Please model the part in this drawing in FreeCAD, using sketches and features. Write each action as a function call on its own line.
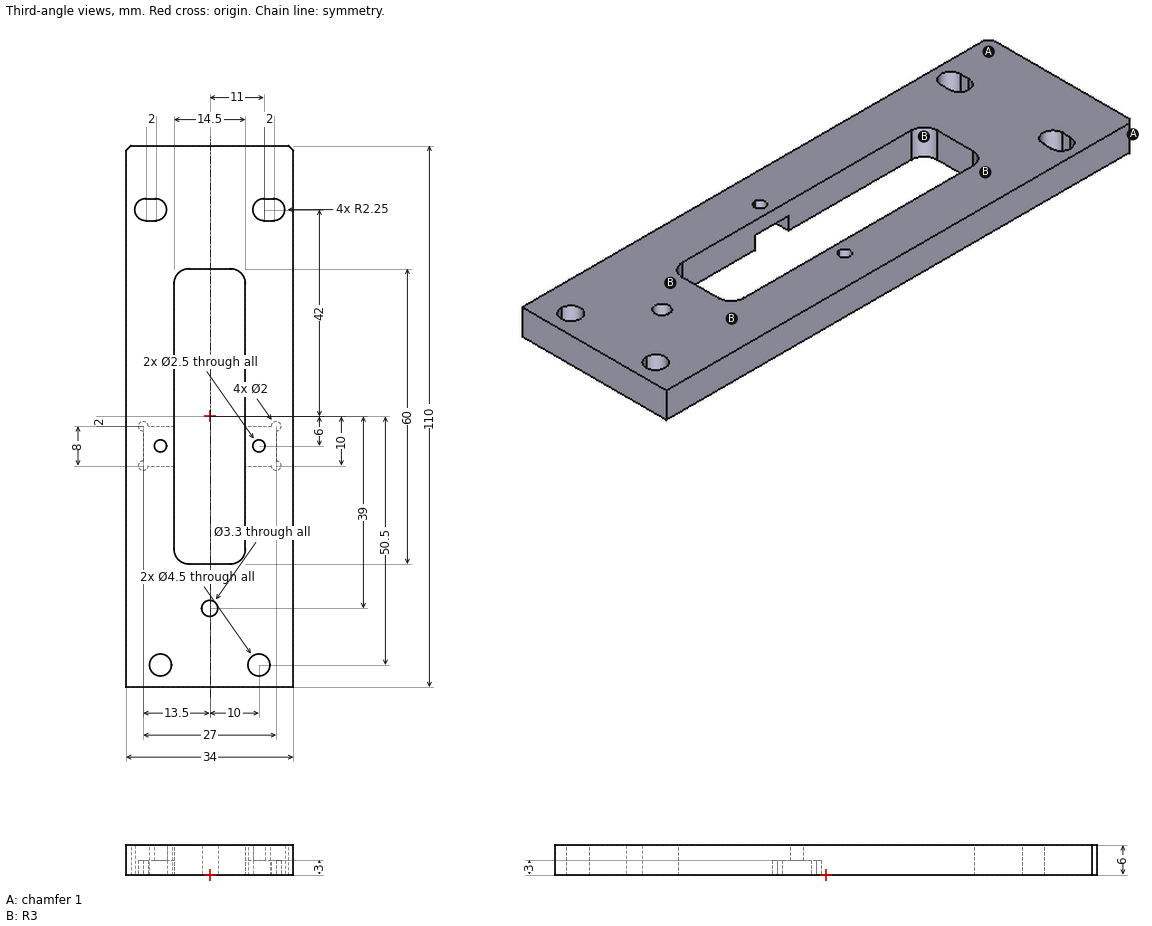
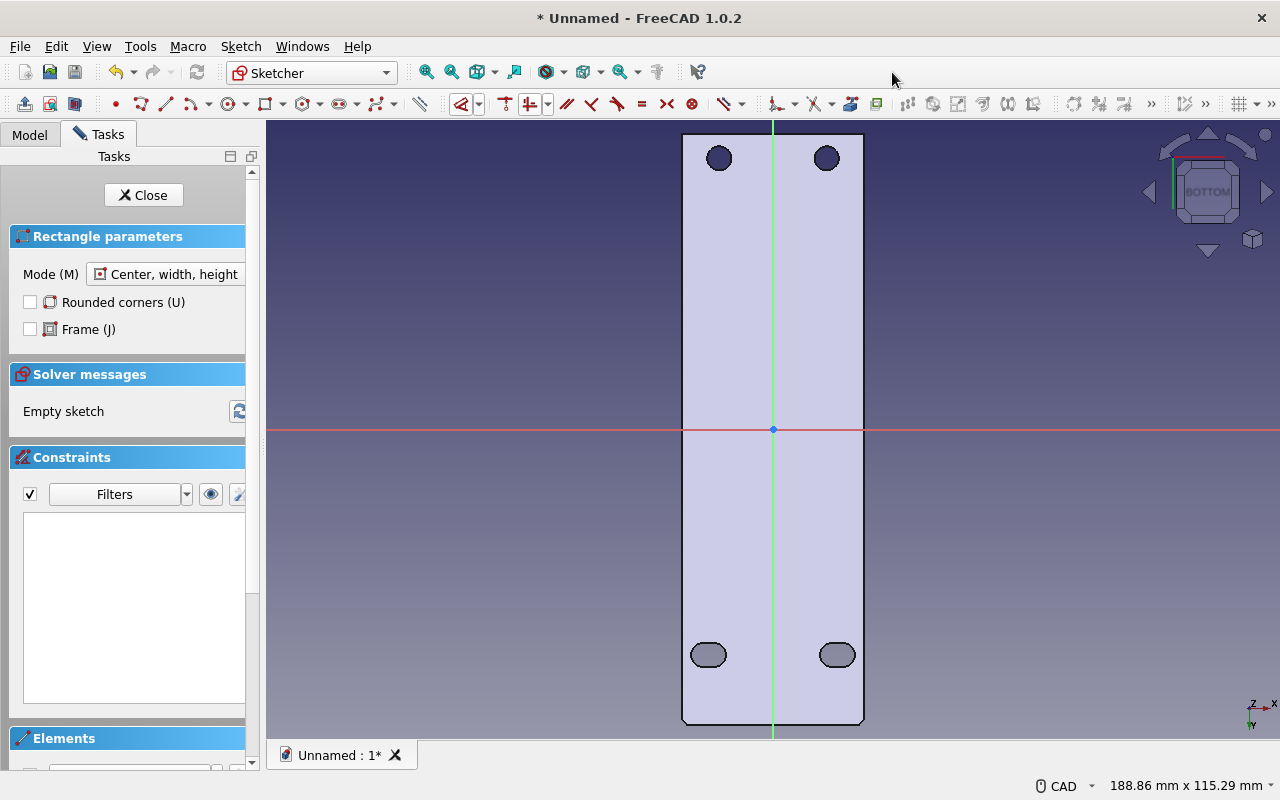
click(773, 430)
click(812, 268)
key(Escape)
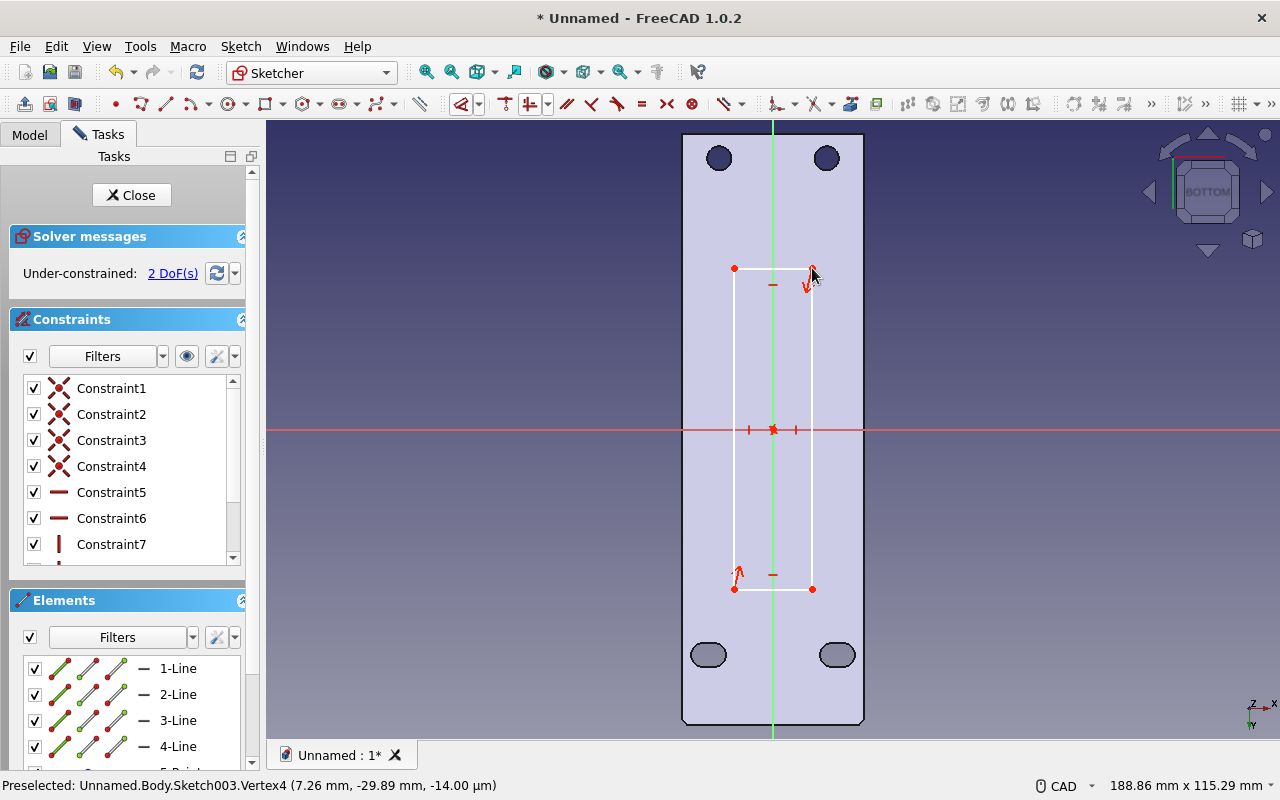
click(812, 494)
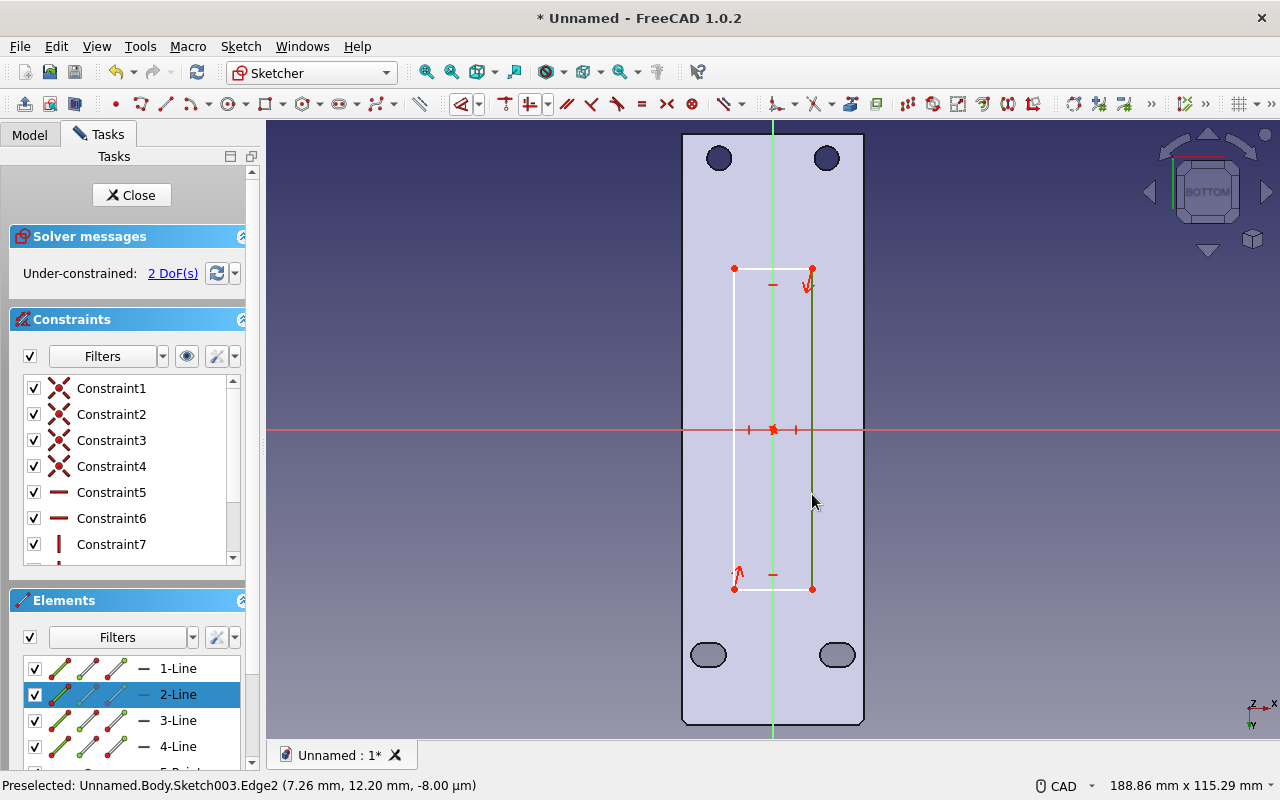
key(i)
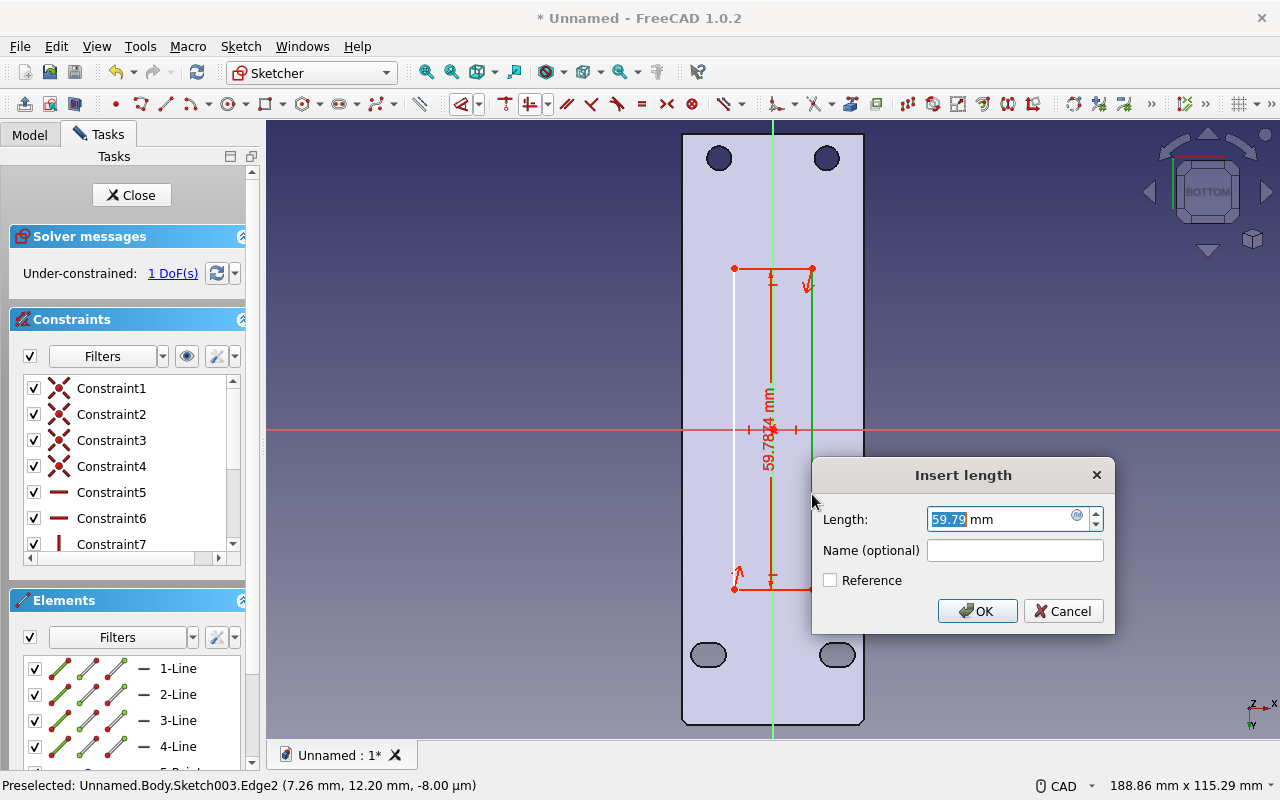
text(60)
key(Return)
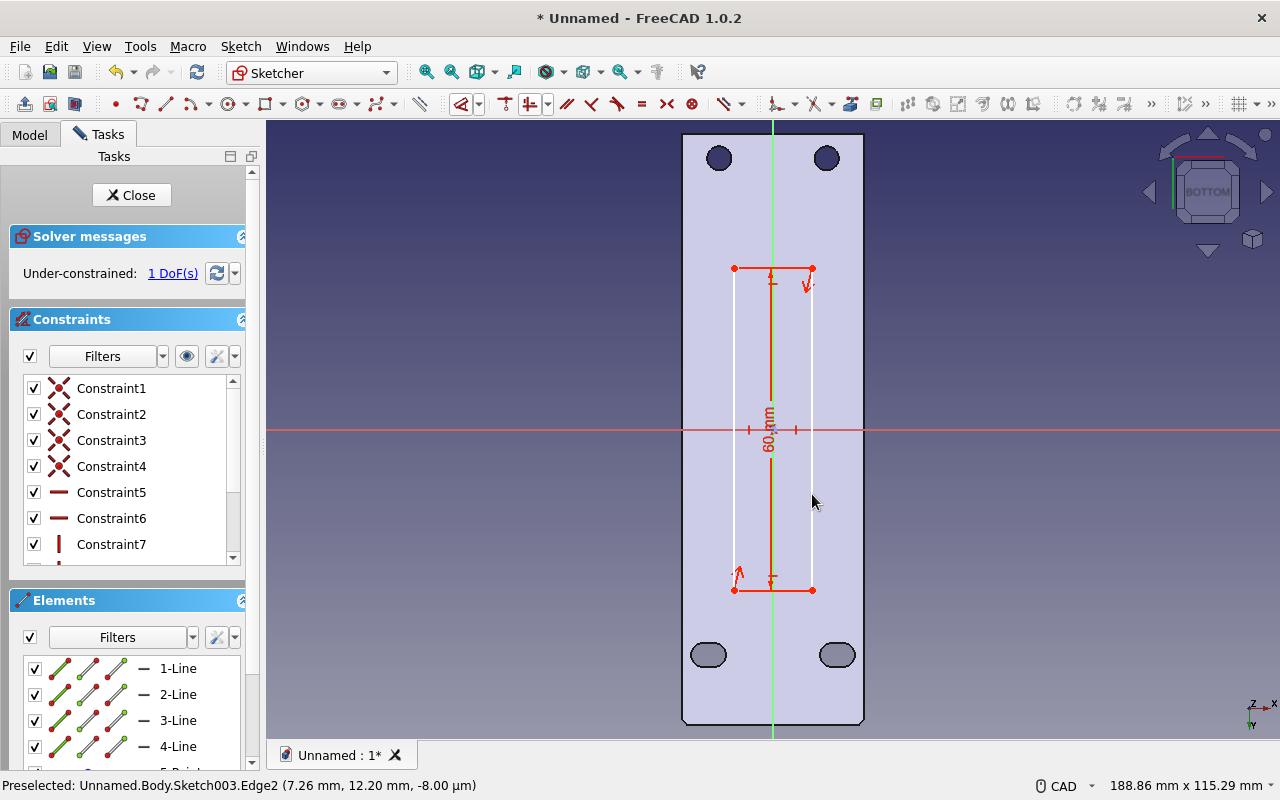
click(757, 591)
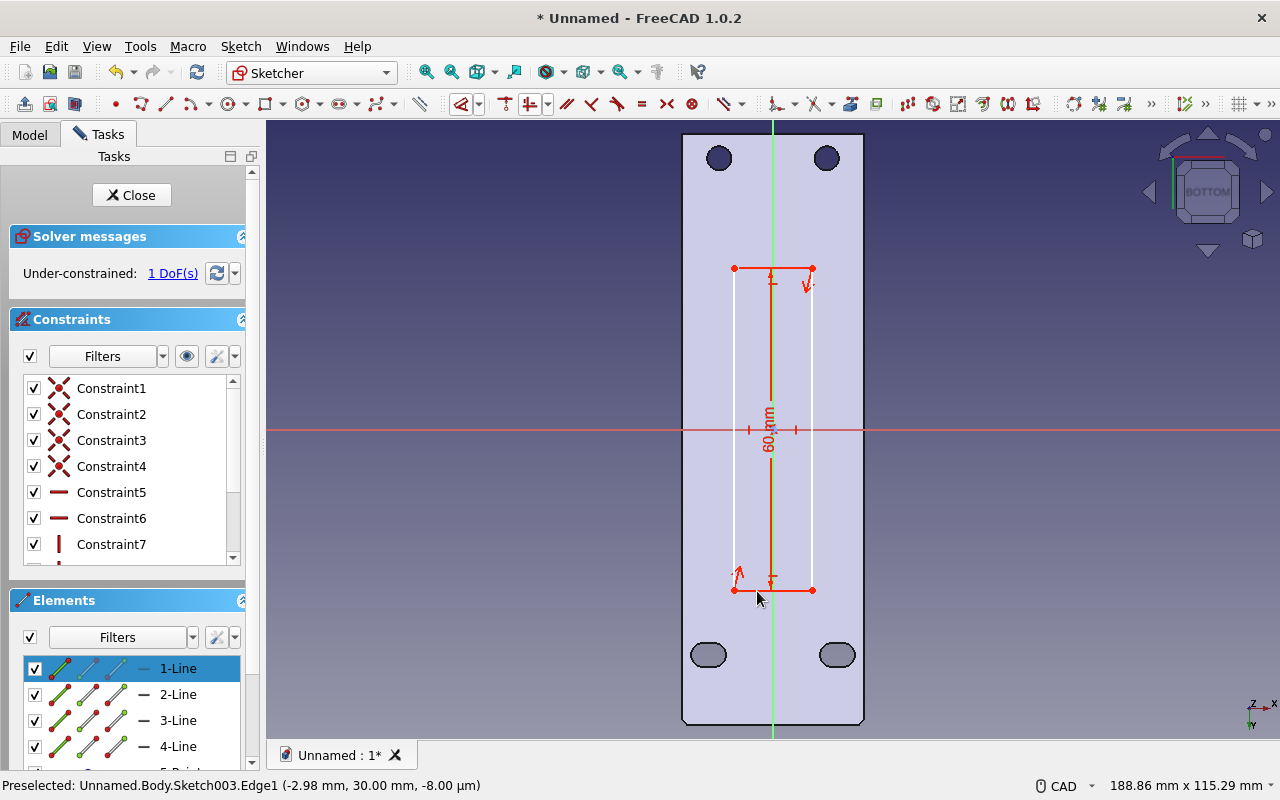
click(478, 104)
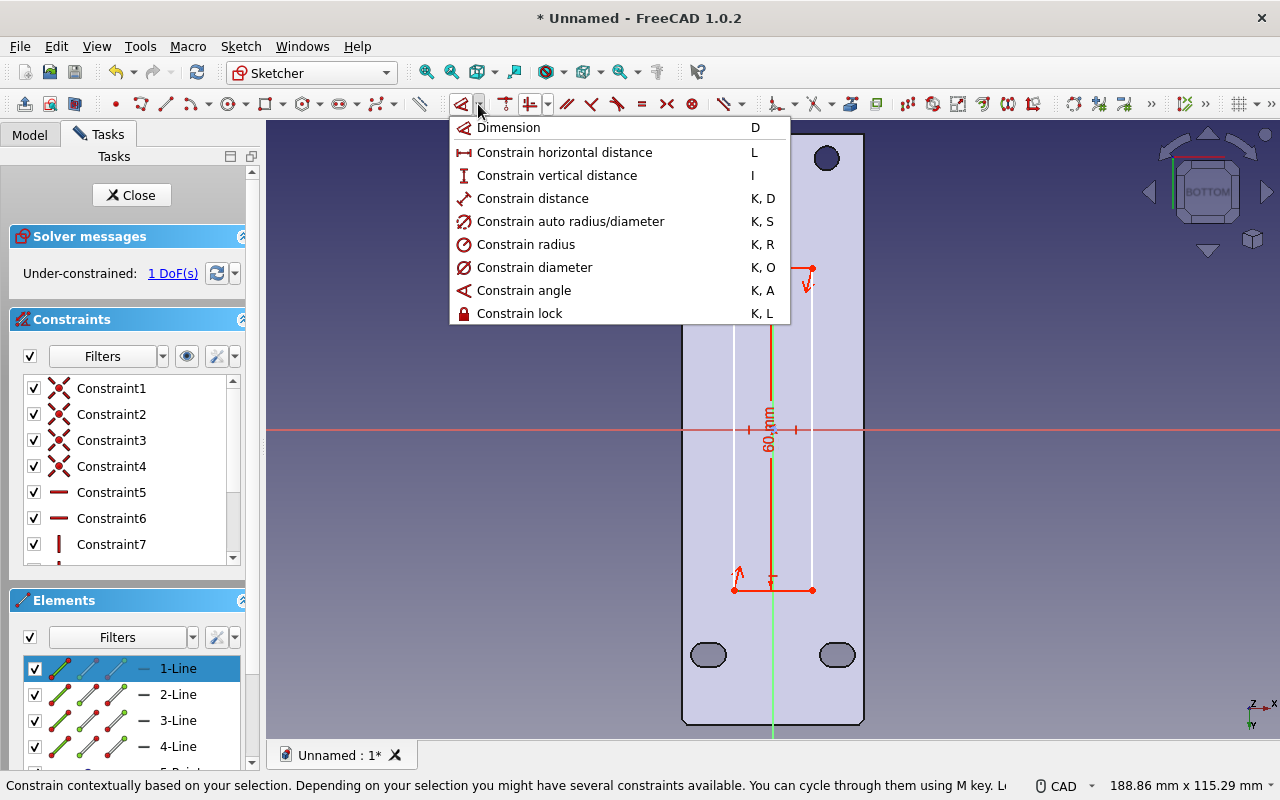
click(620, 152)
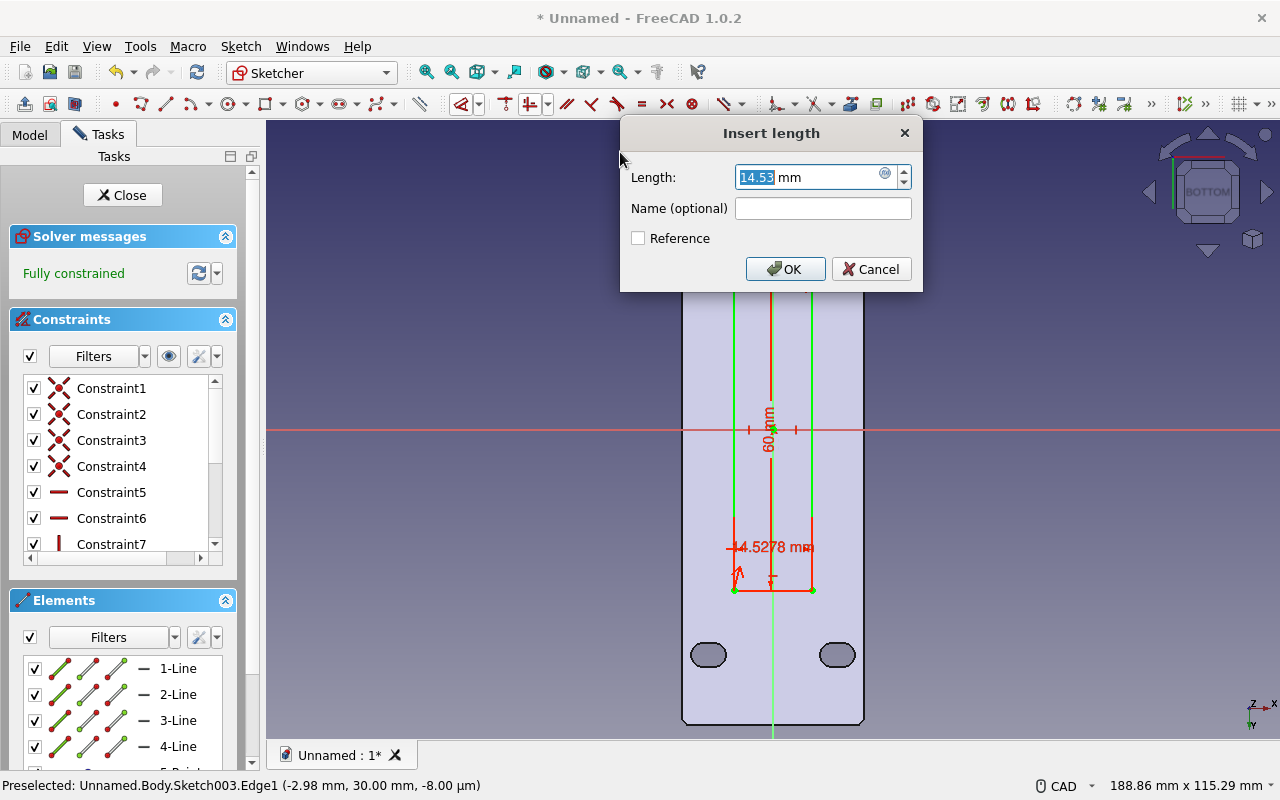
text(14.5)
key(Return)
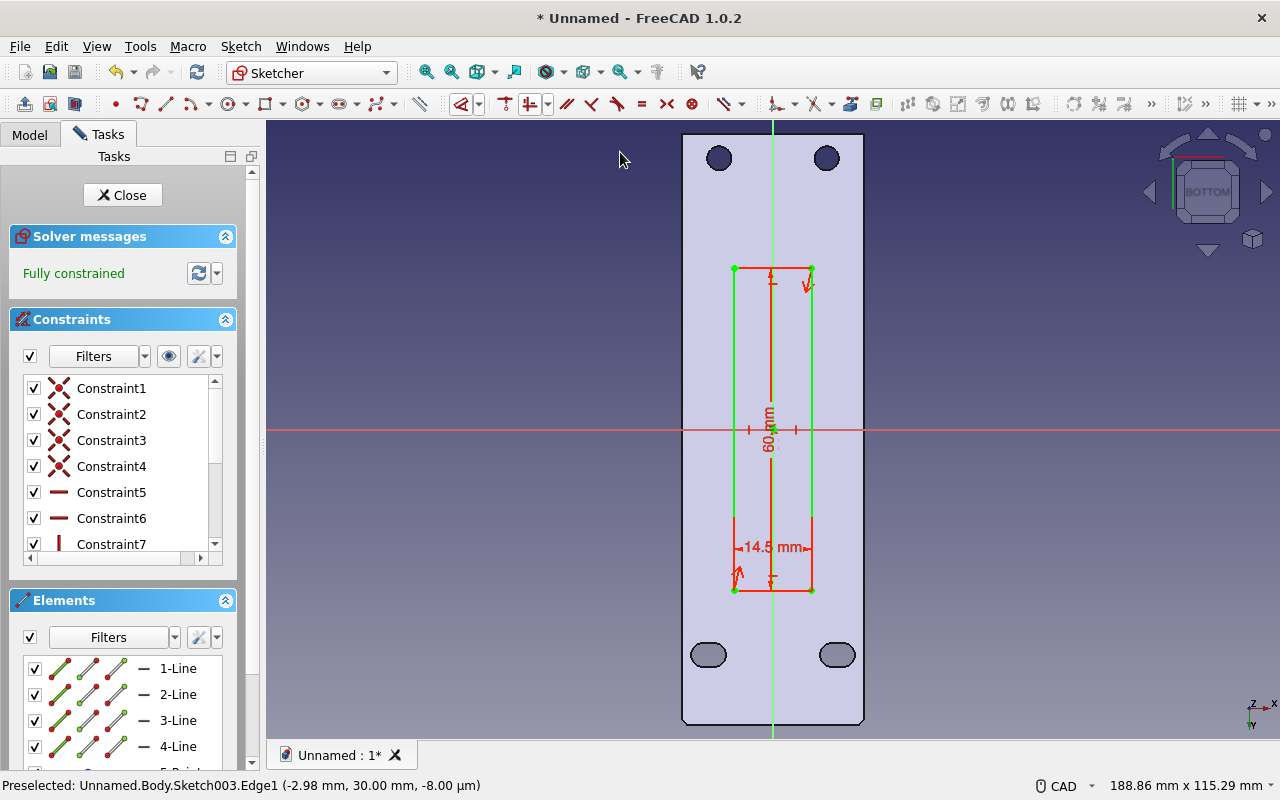
click(123, 195)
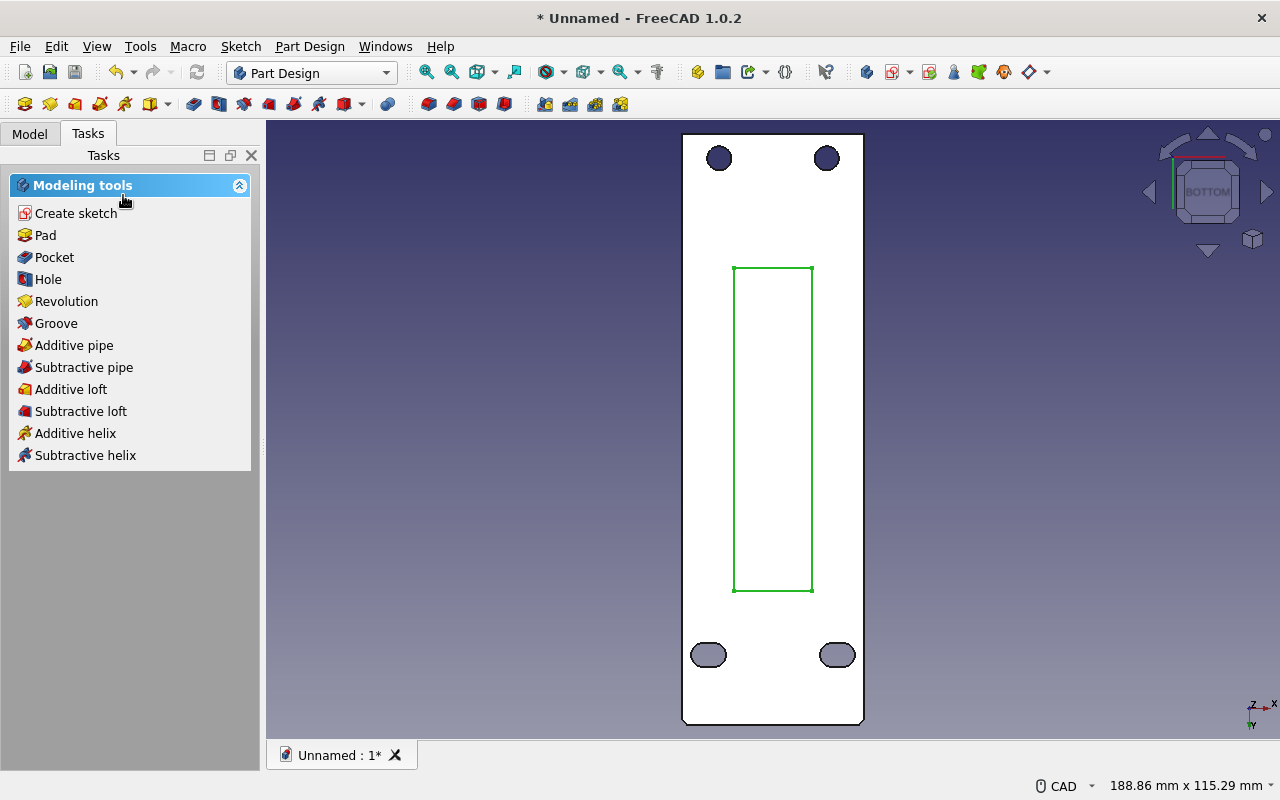
click(194, 104)